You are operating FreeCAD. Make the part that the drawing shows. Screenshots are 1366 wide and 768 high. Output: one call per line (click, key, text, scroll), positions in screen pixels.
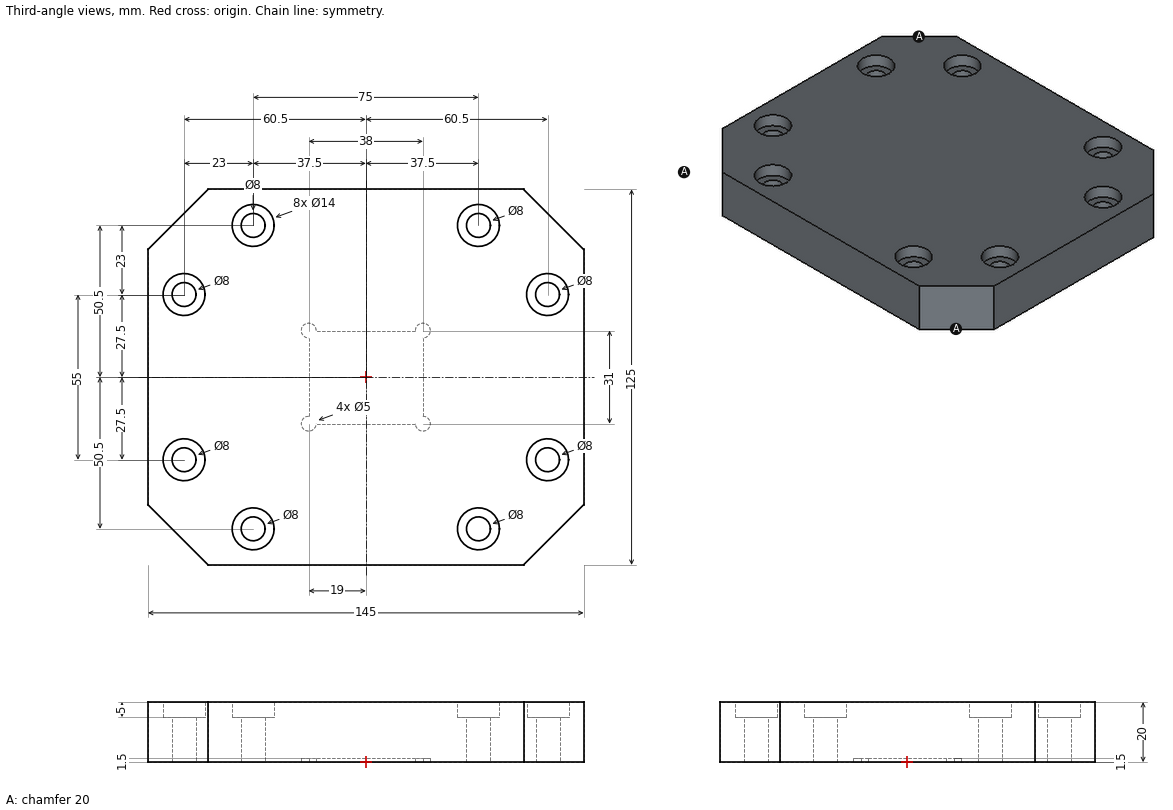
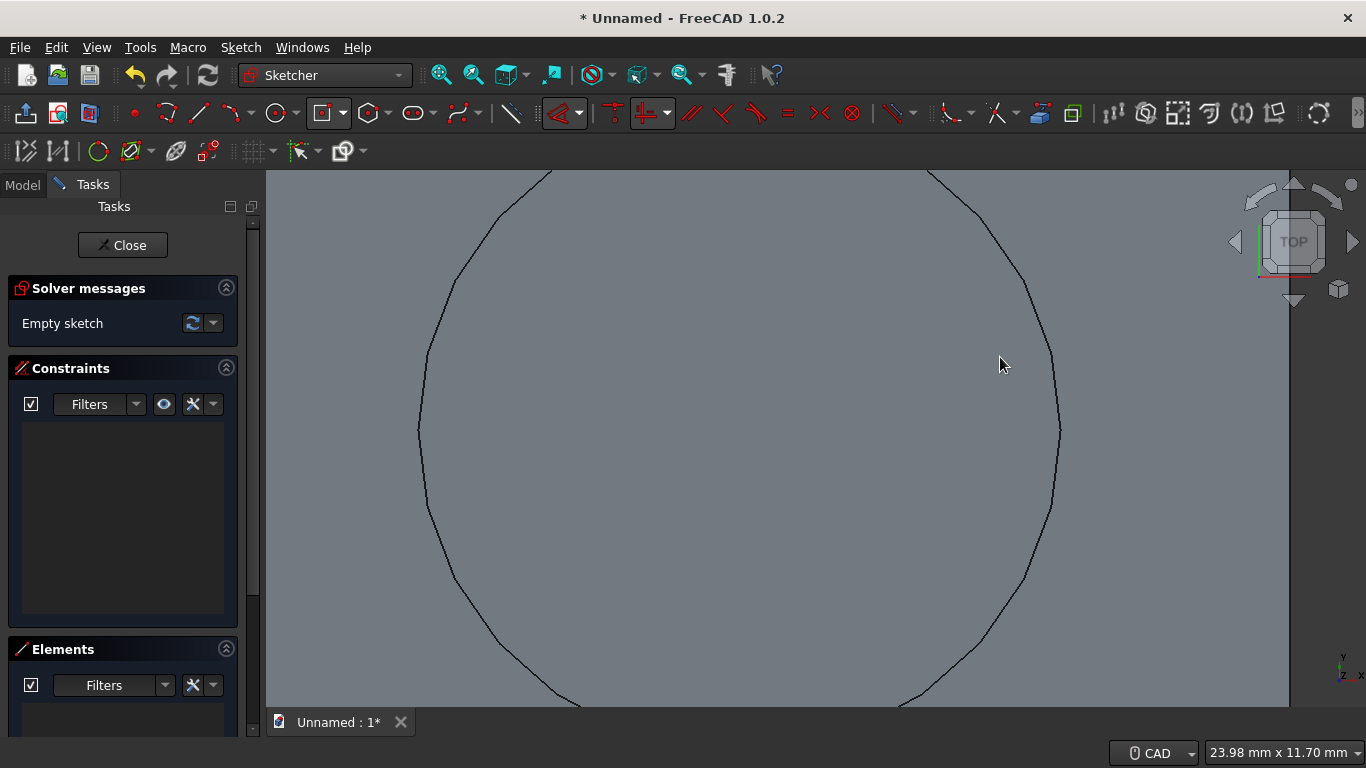
click(276, 114)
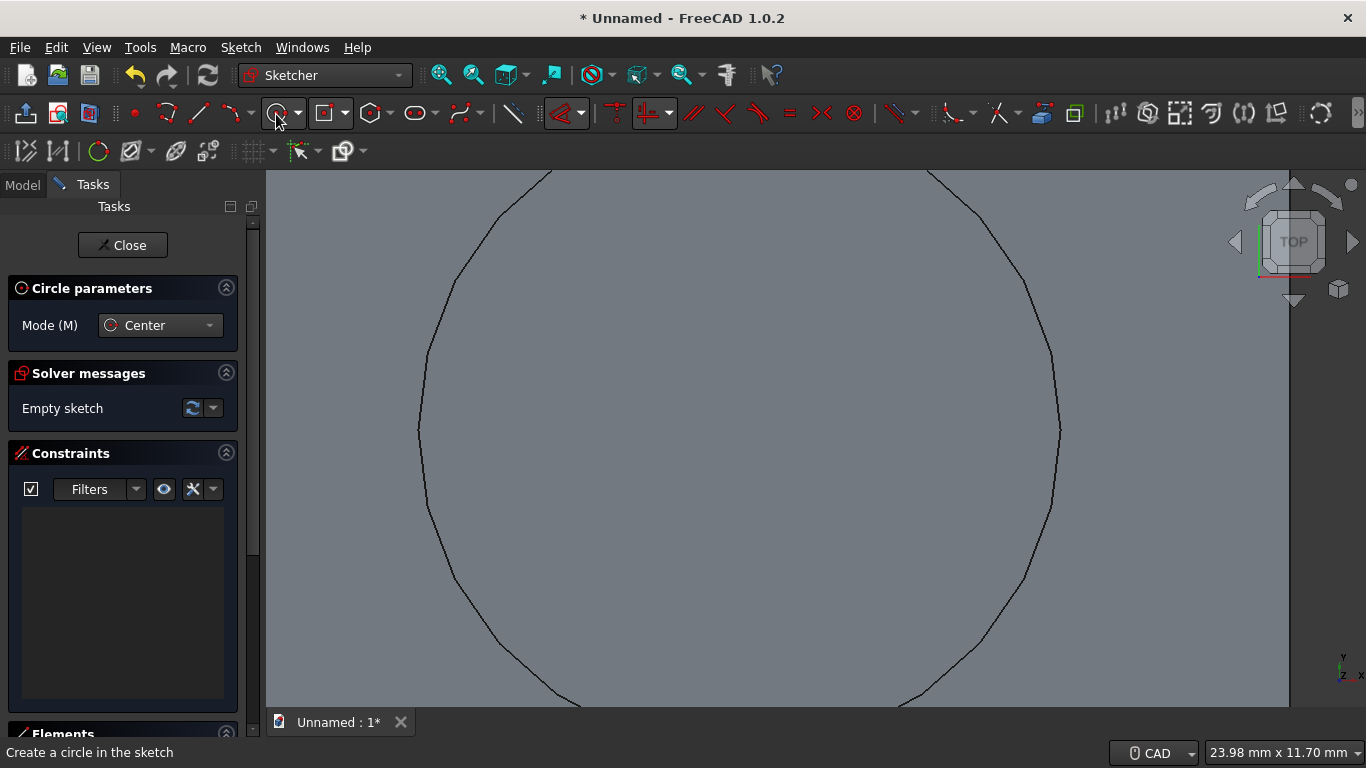
click(739, 430)
click(869, 300)
key(Escape)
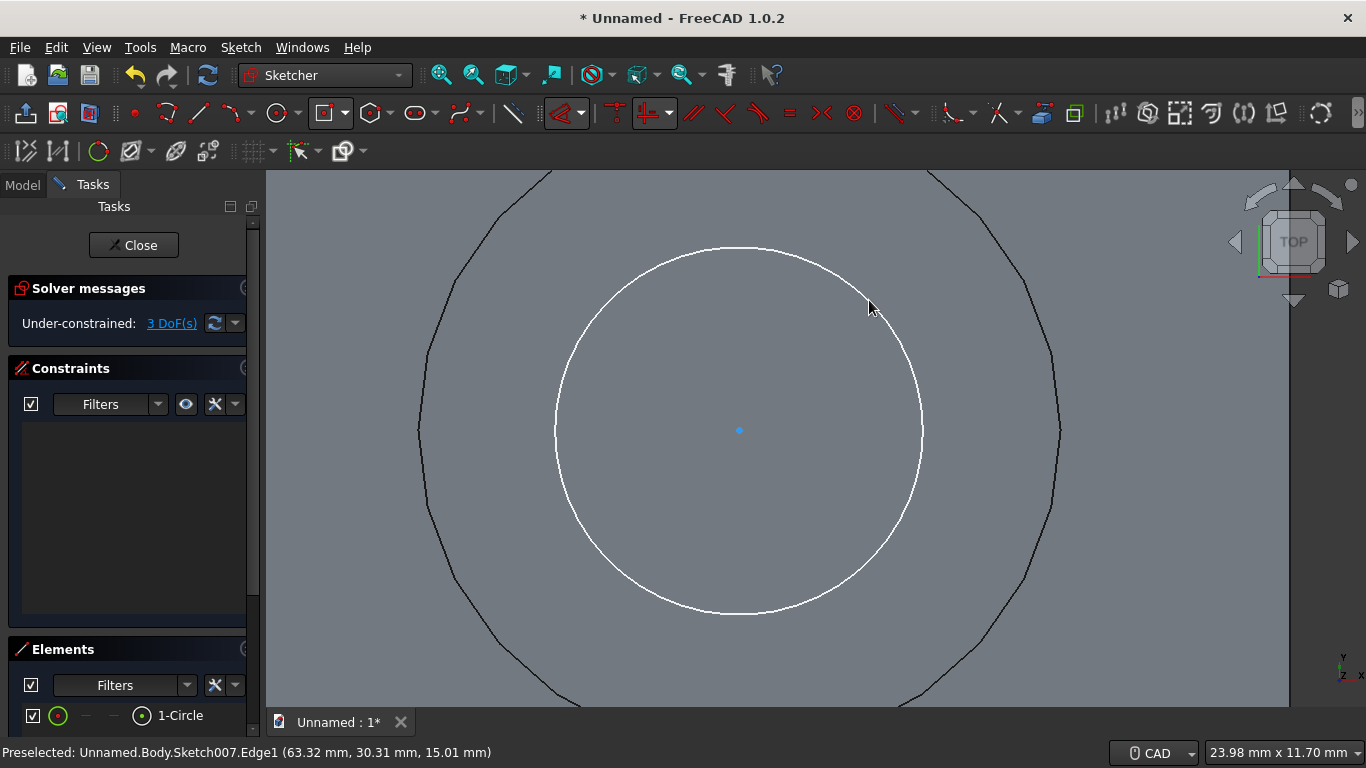
click(869, 301)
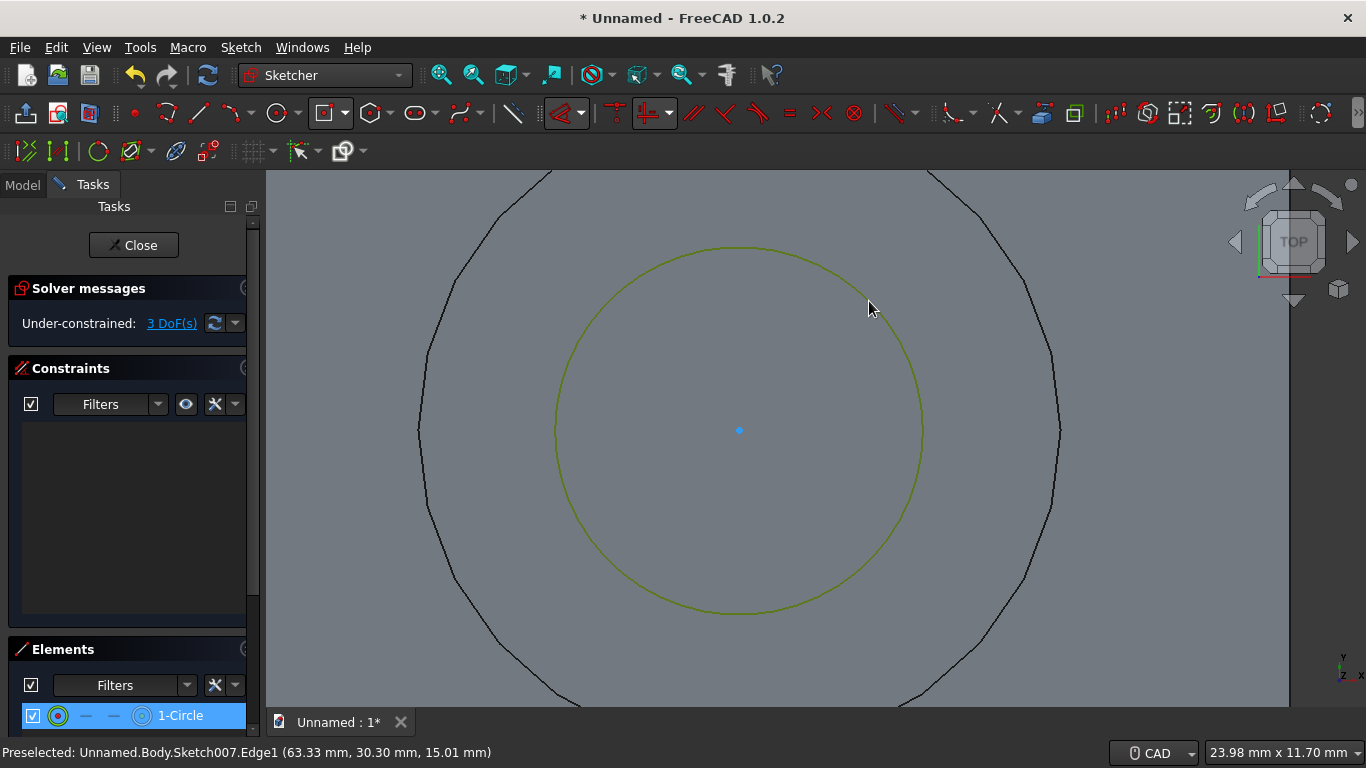
key(k)
key(o)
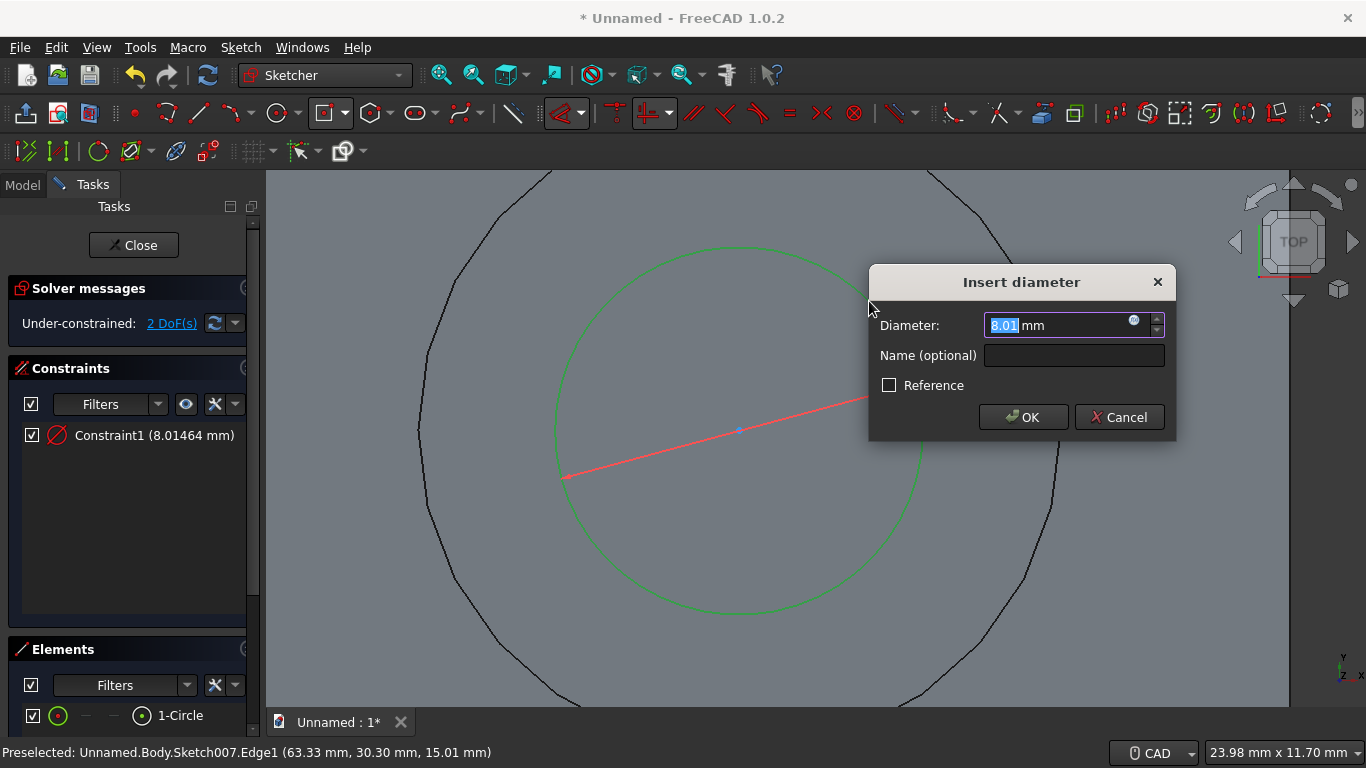
text(8)
key(Return)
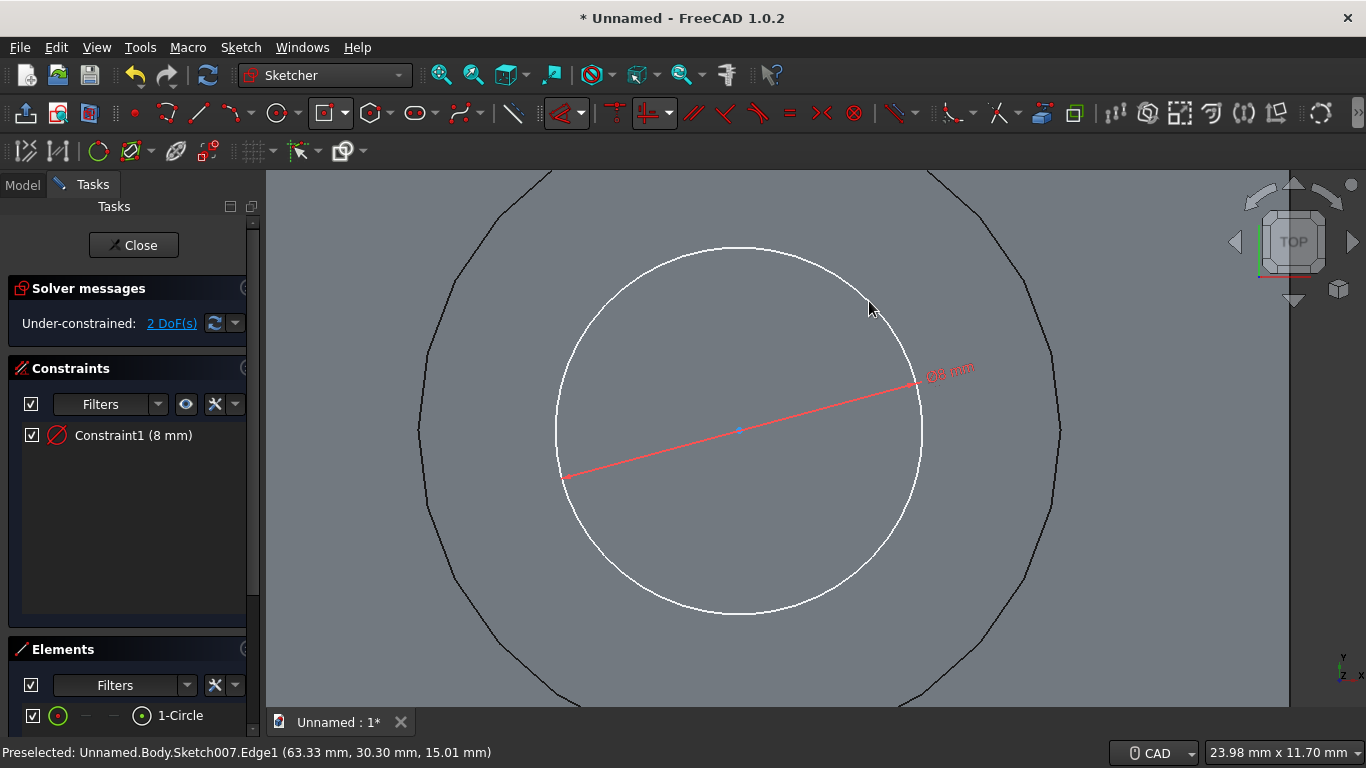
click(739, 431)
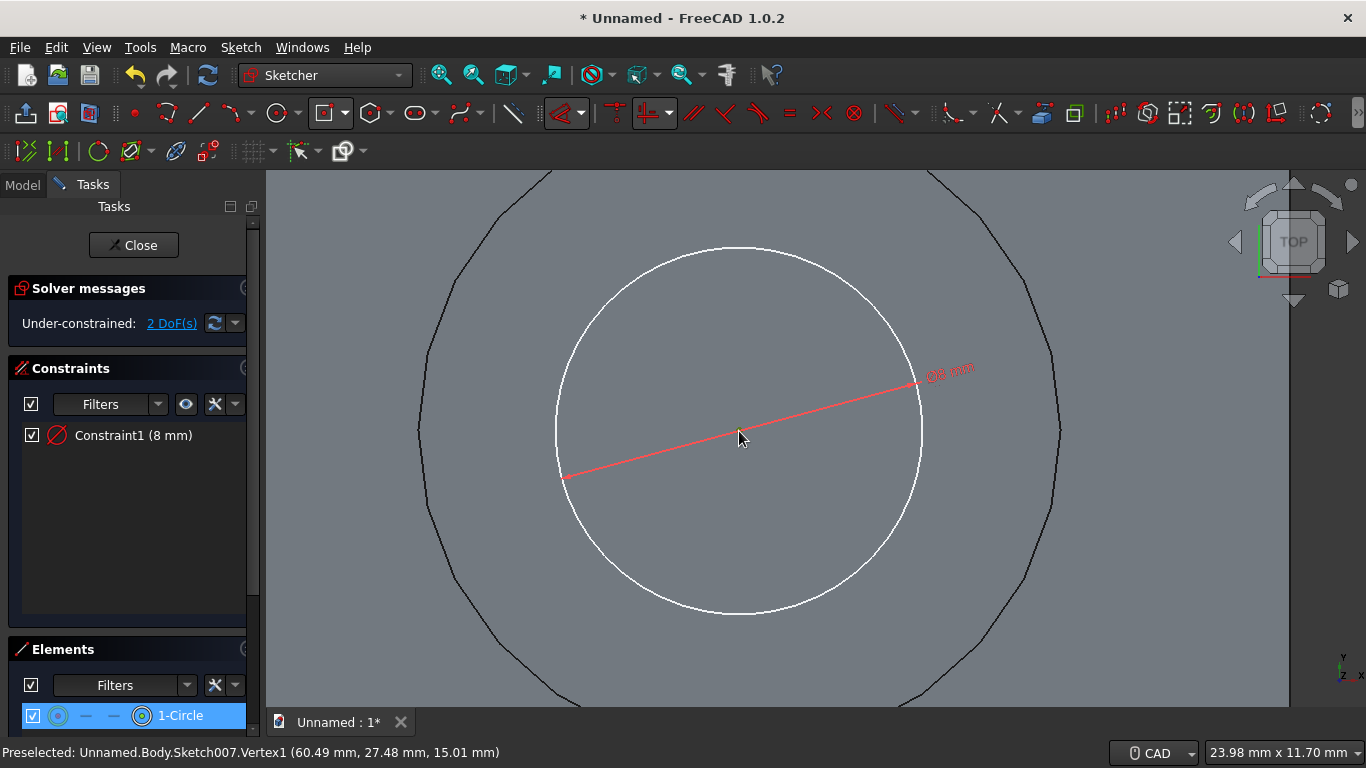
key(l)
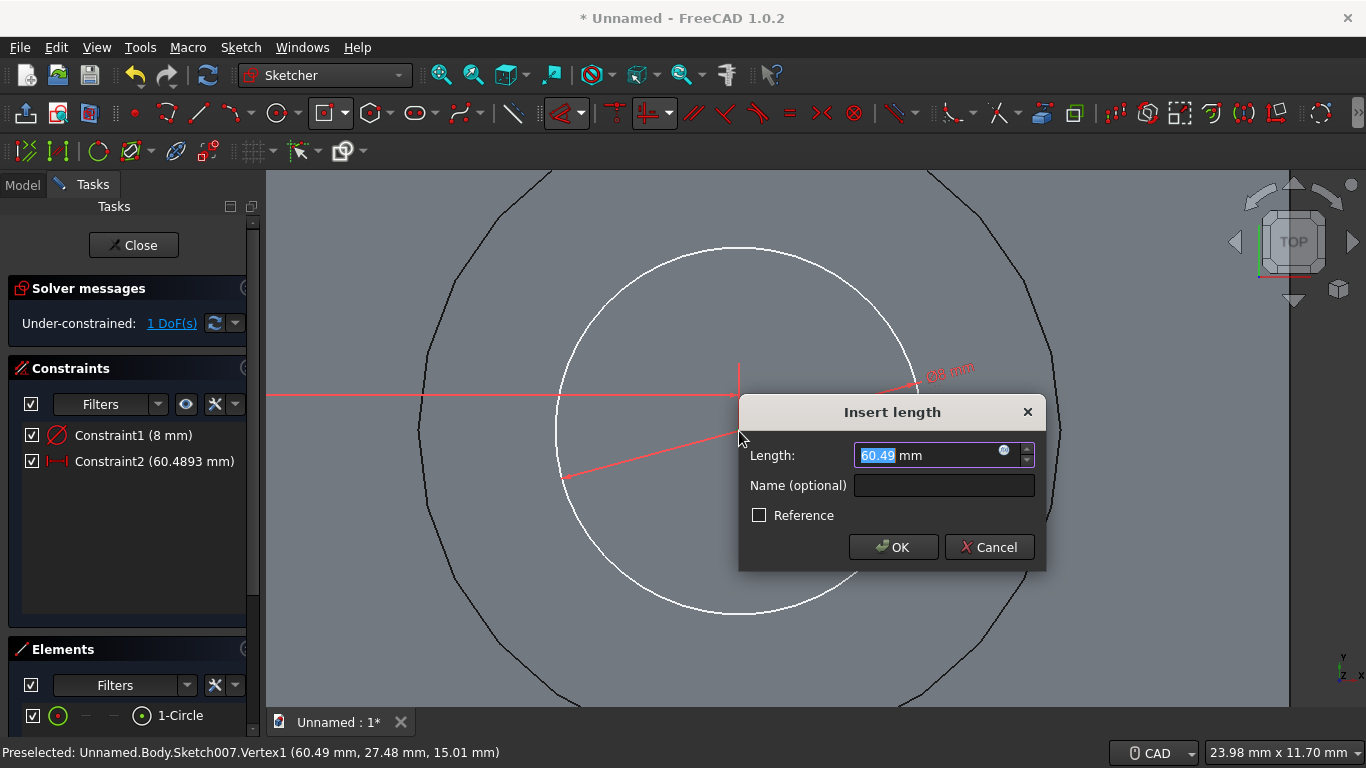
text(60.5)
key(Return)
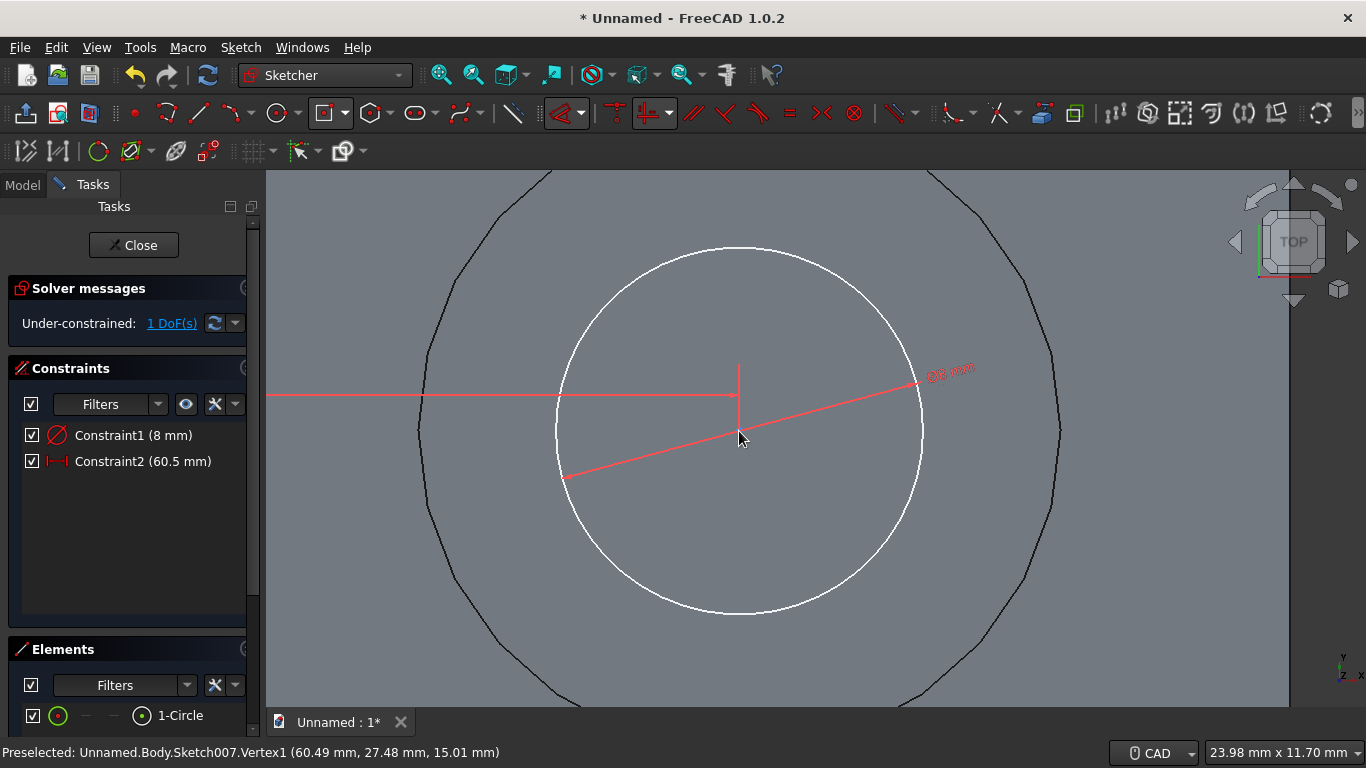
click(739, 431)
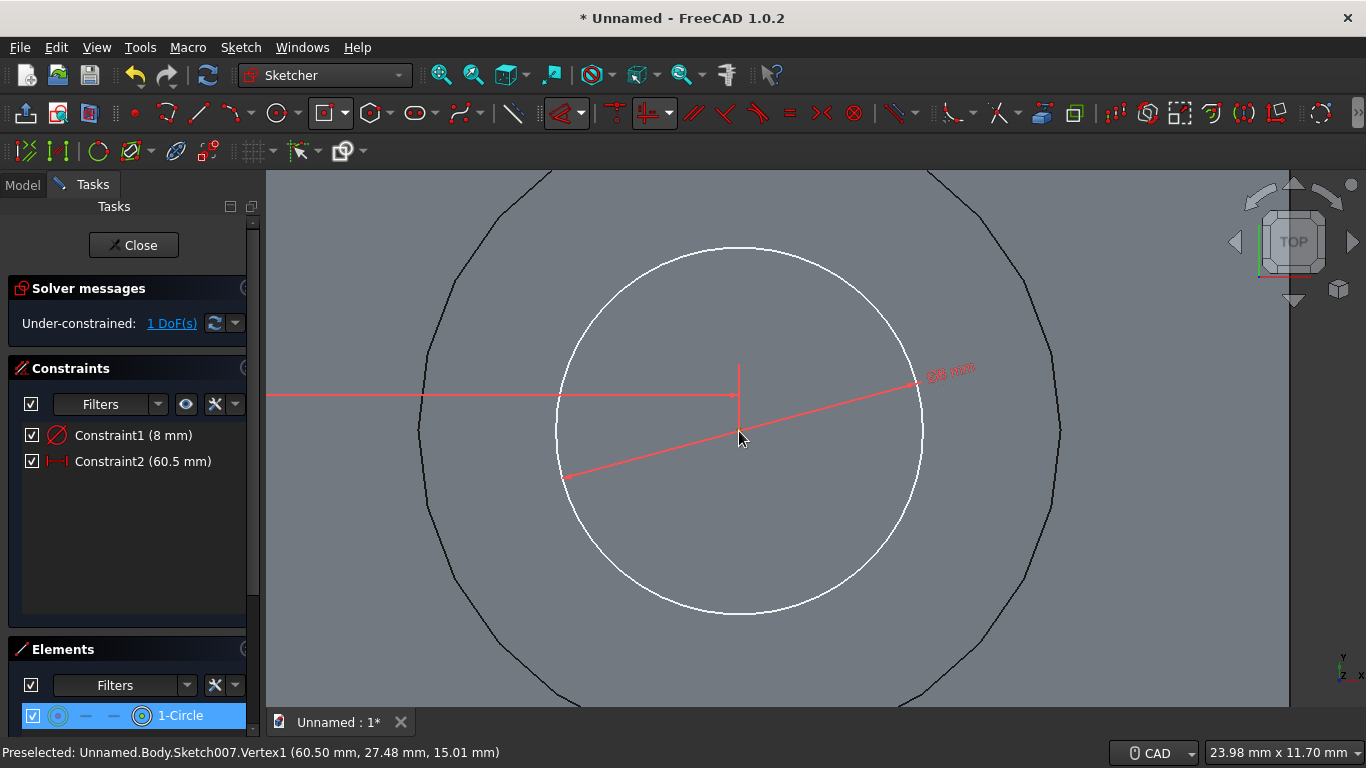
key(i)